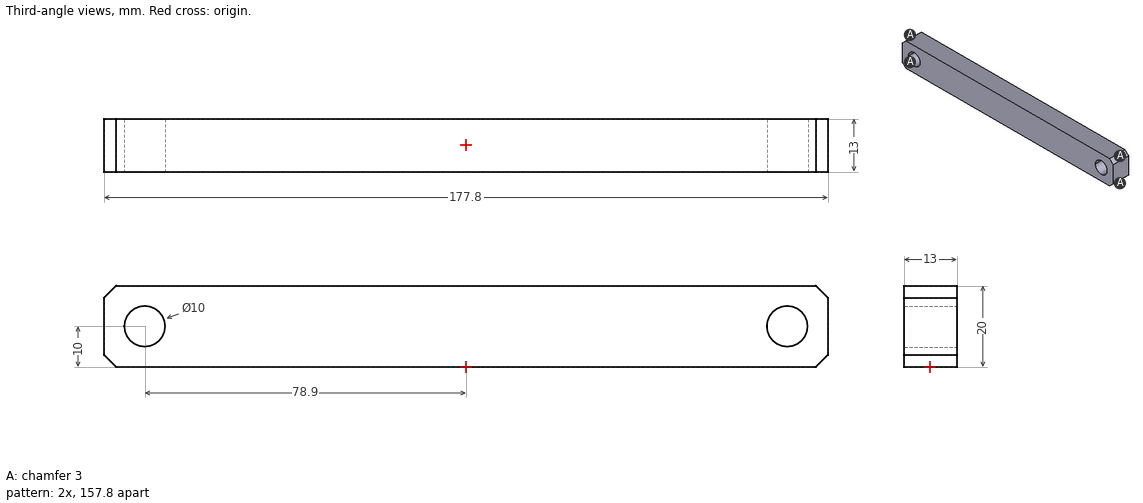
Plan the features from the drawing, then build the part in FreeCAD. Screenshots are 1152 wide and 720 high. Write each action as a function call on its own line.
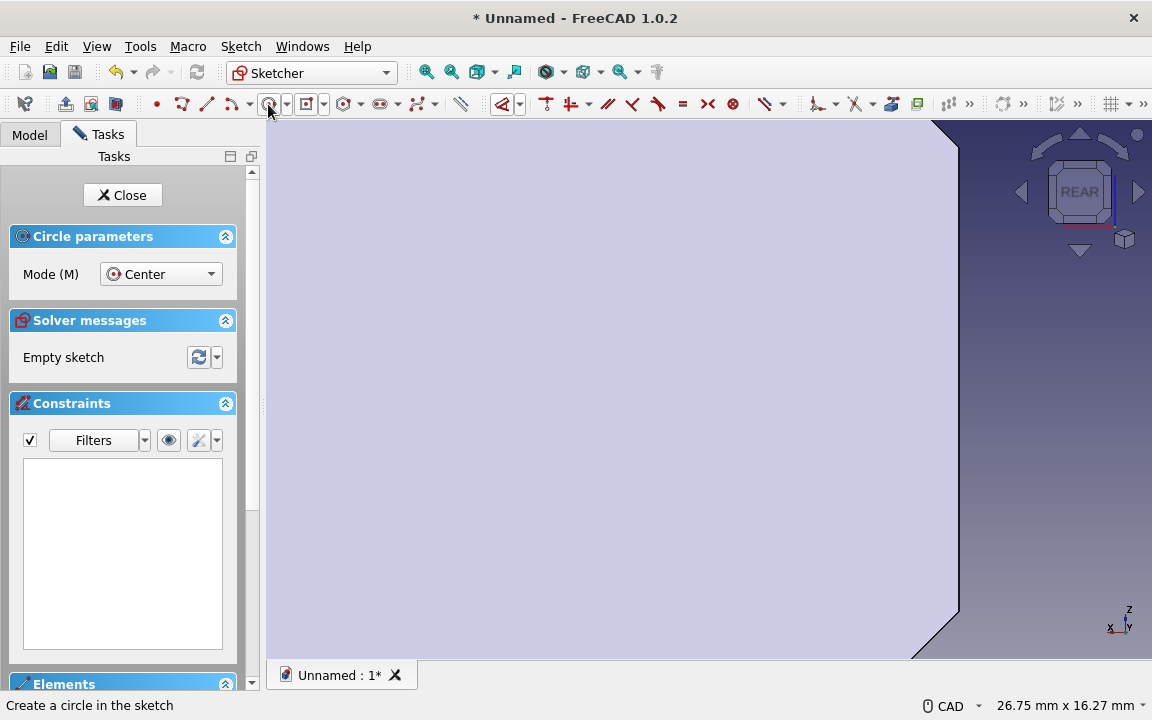
click(628, 379)
click(745, 262)
key(Escape)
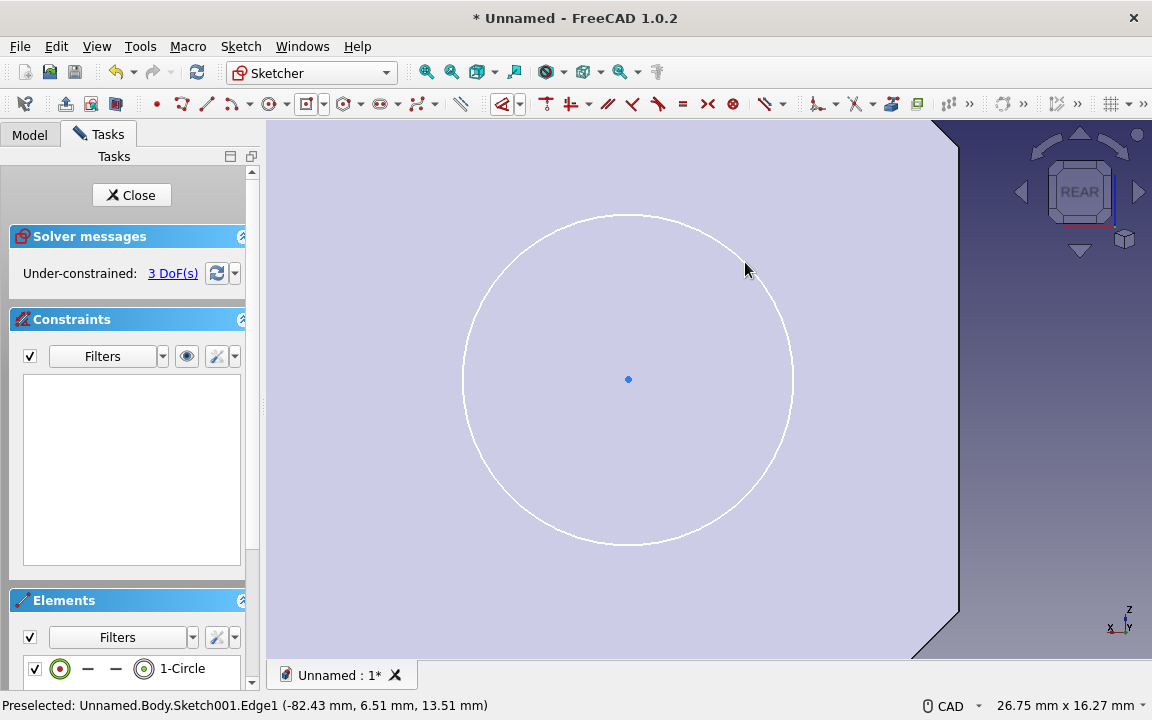
click(745, 263)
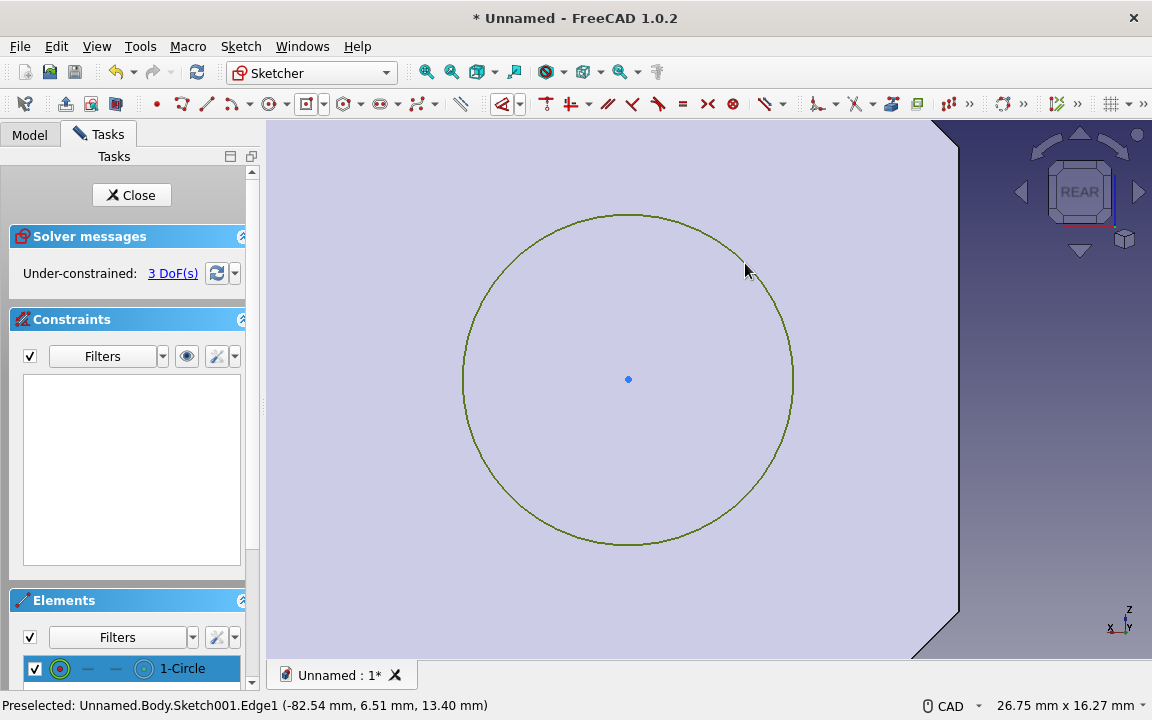
key(k)
key(o)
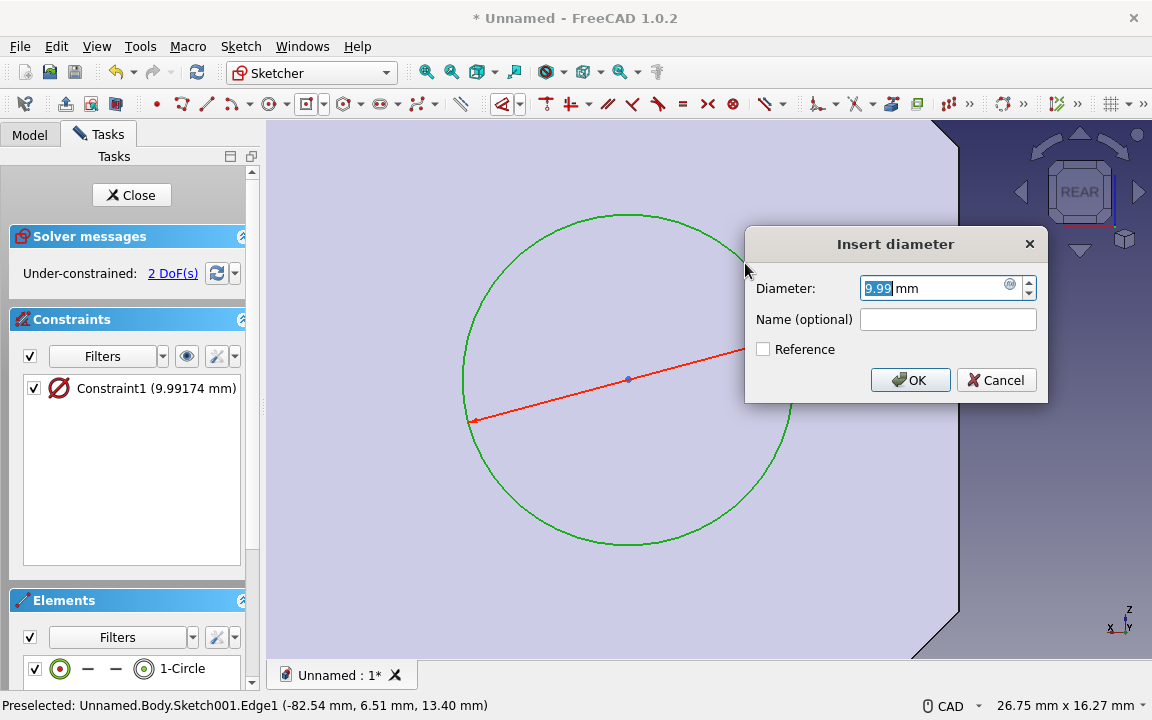
text(10)
key(Return)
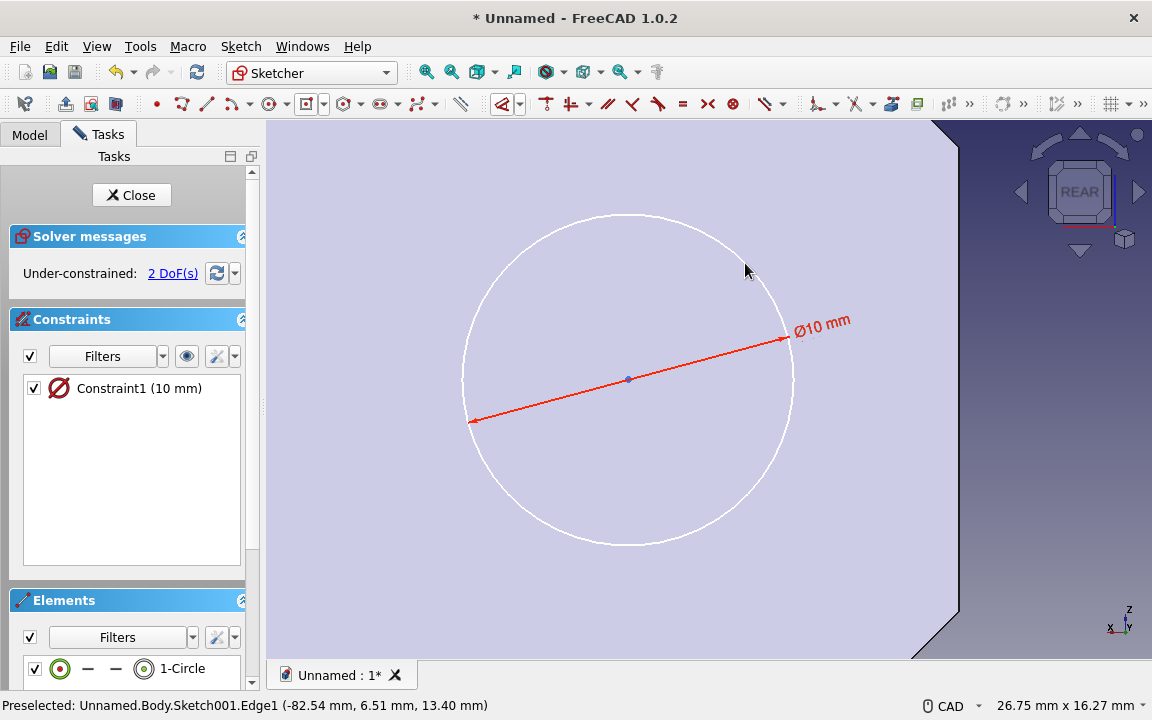
click(628, 380)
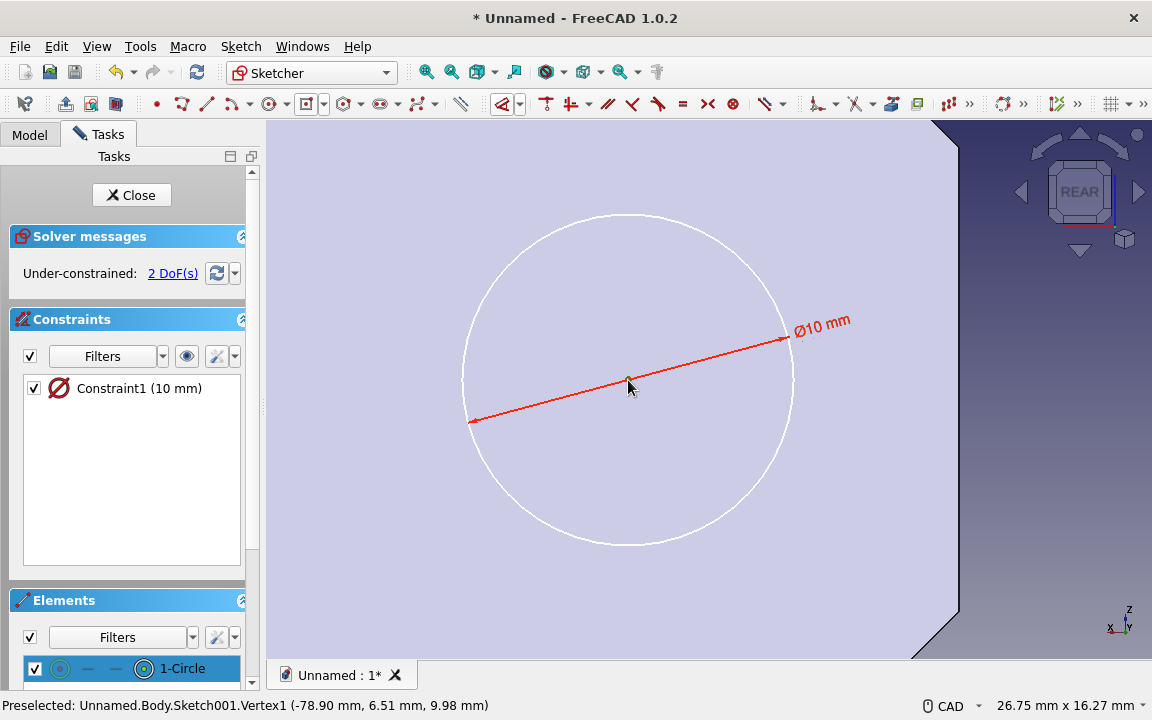
click(520, 104)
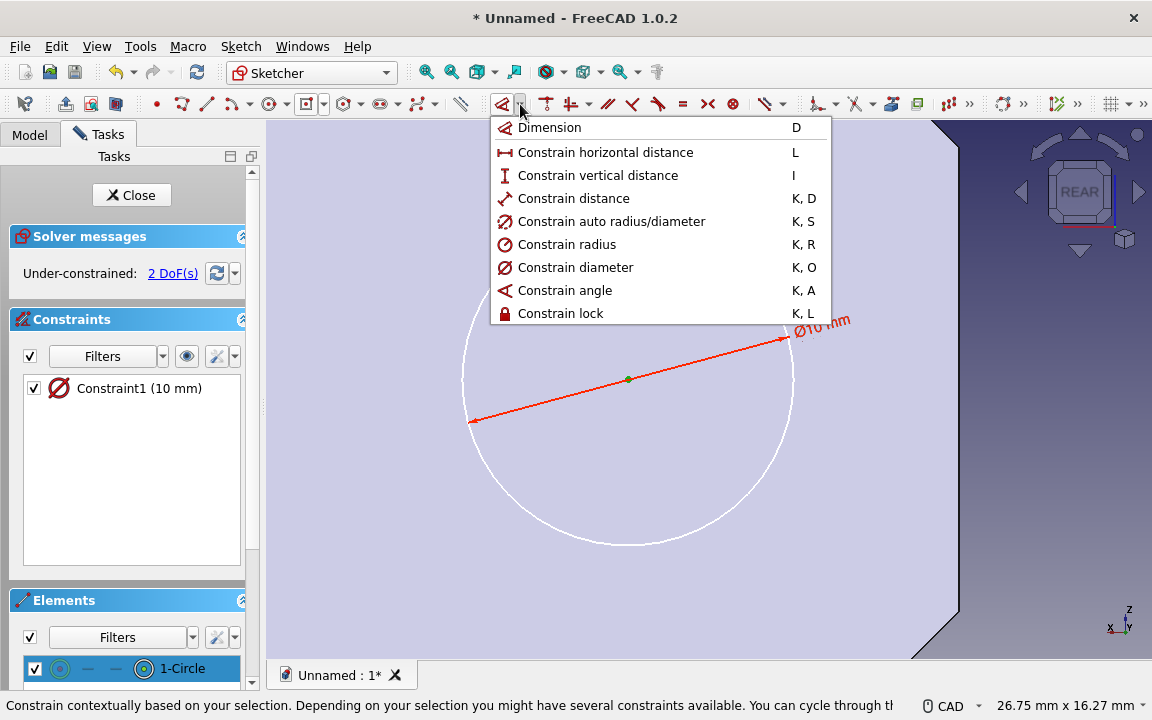
click(661, 176)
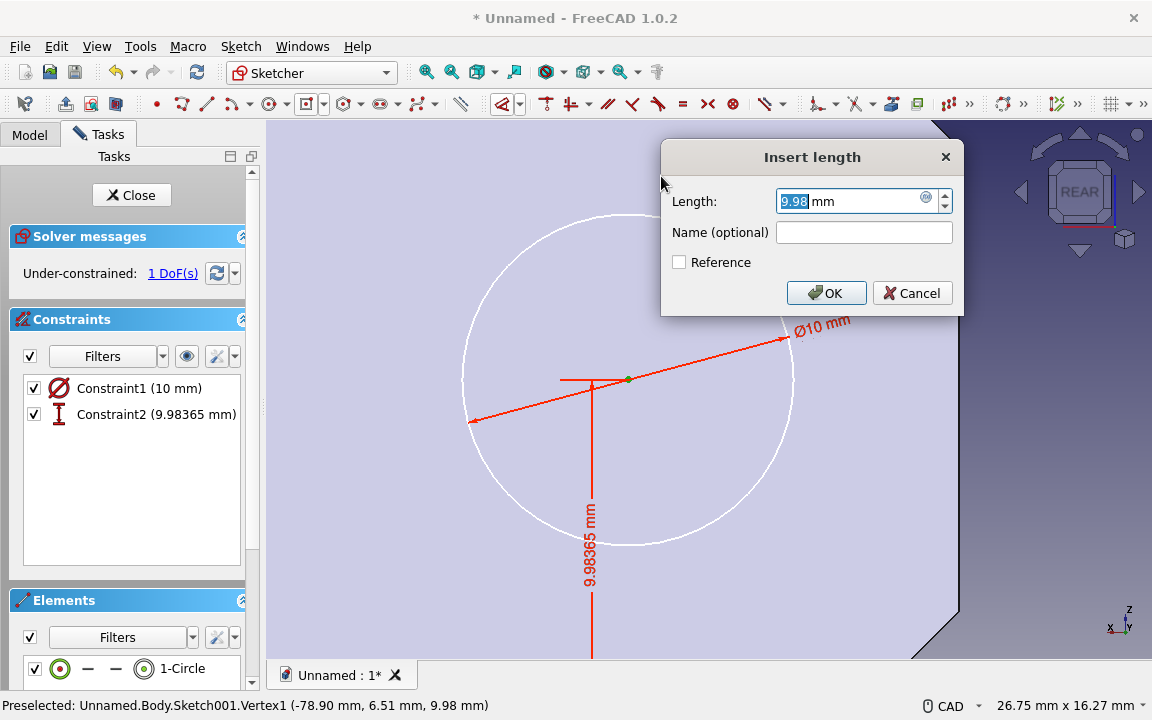
text(10)
key(Return)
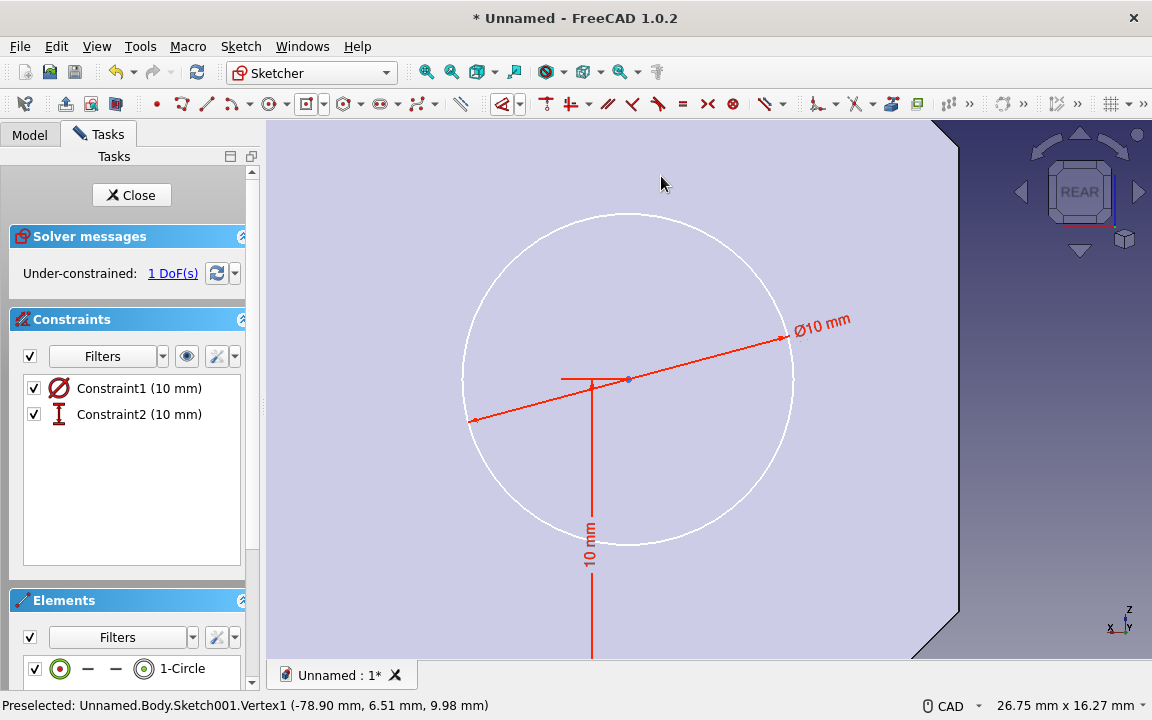
click(628, 379)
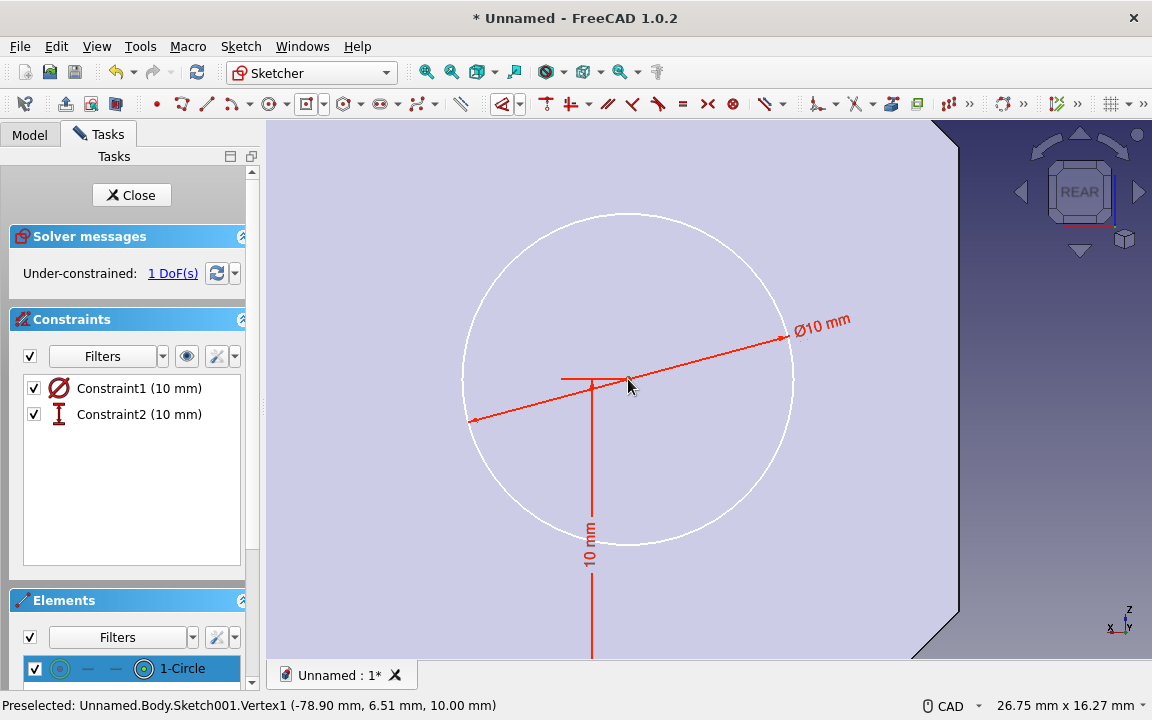
key(l)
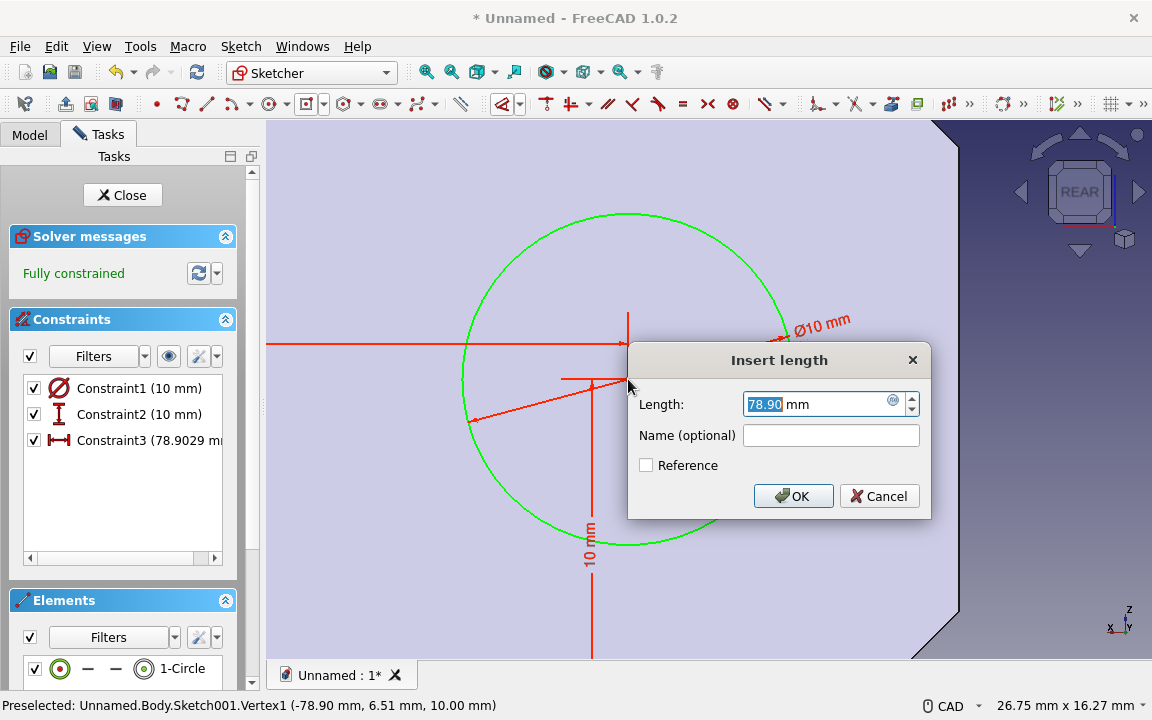
text(78.9)
key(Return)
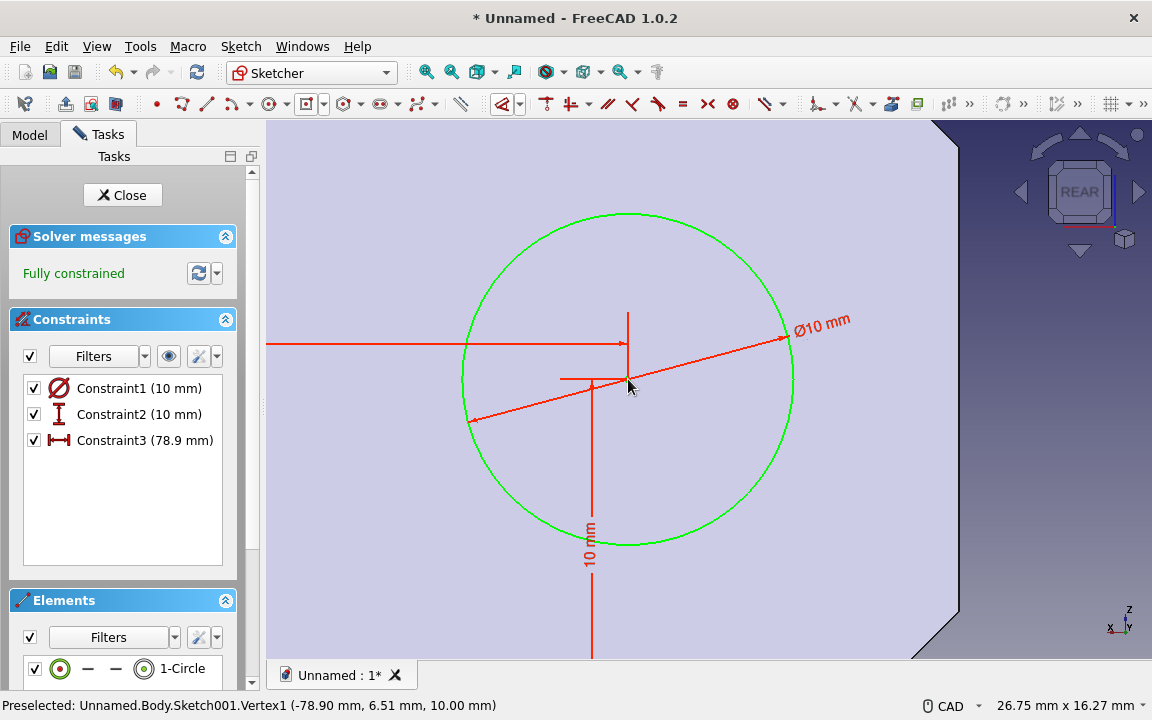
click(123, 195)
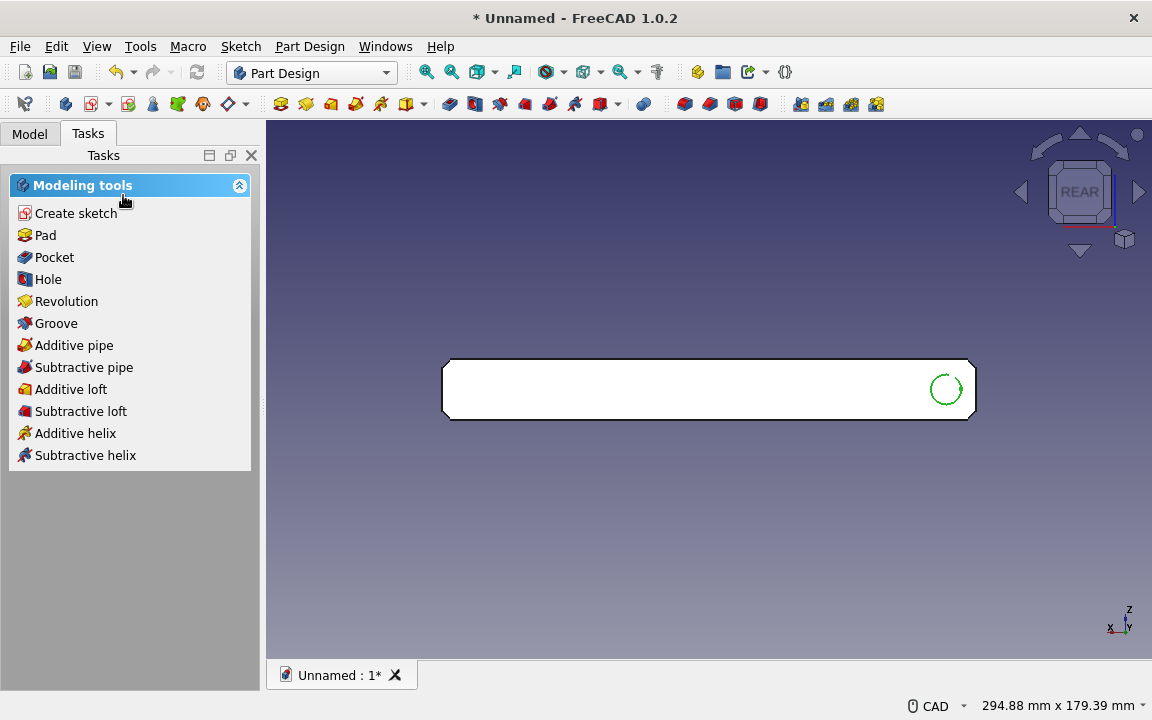
click(450, 104)